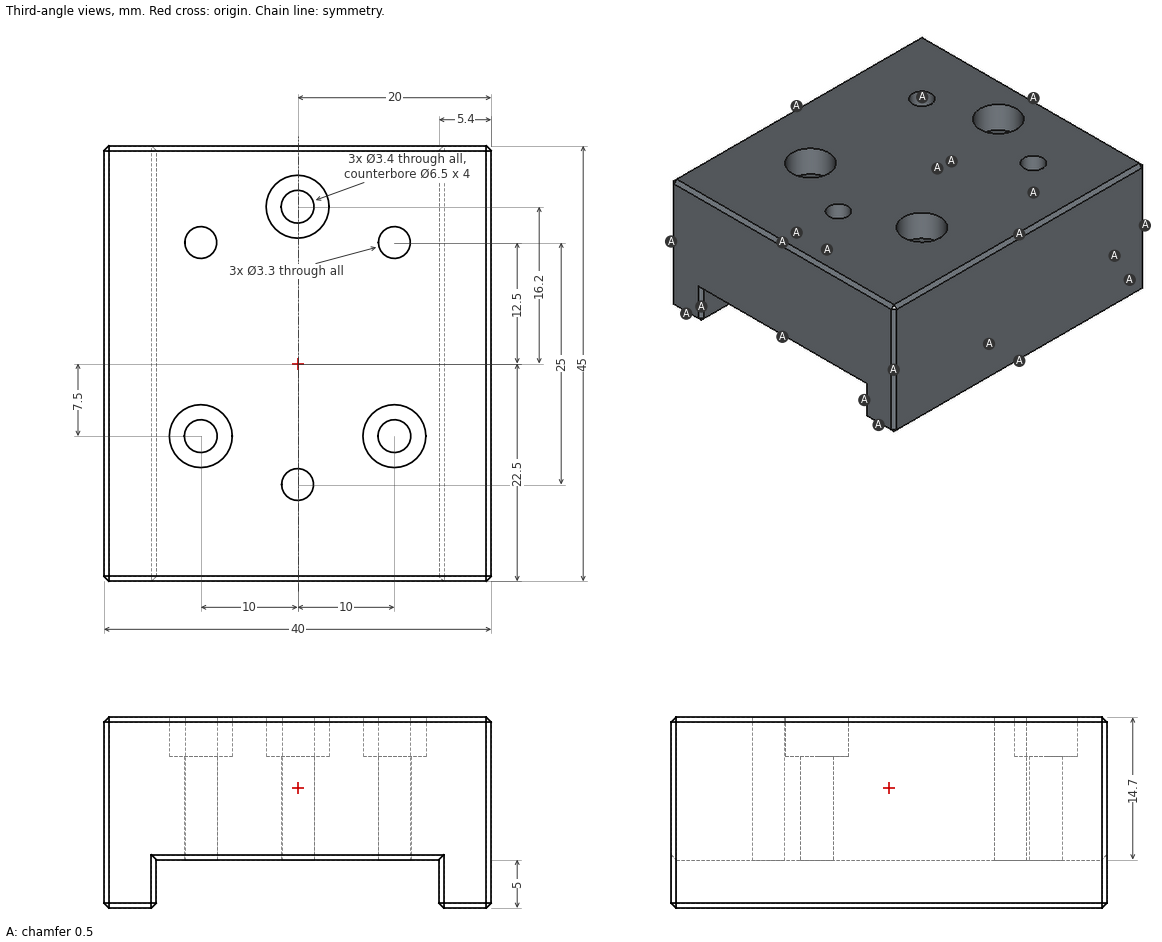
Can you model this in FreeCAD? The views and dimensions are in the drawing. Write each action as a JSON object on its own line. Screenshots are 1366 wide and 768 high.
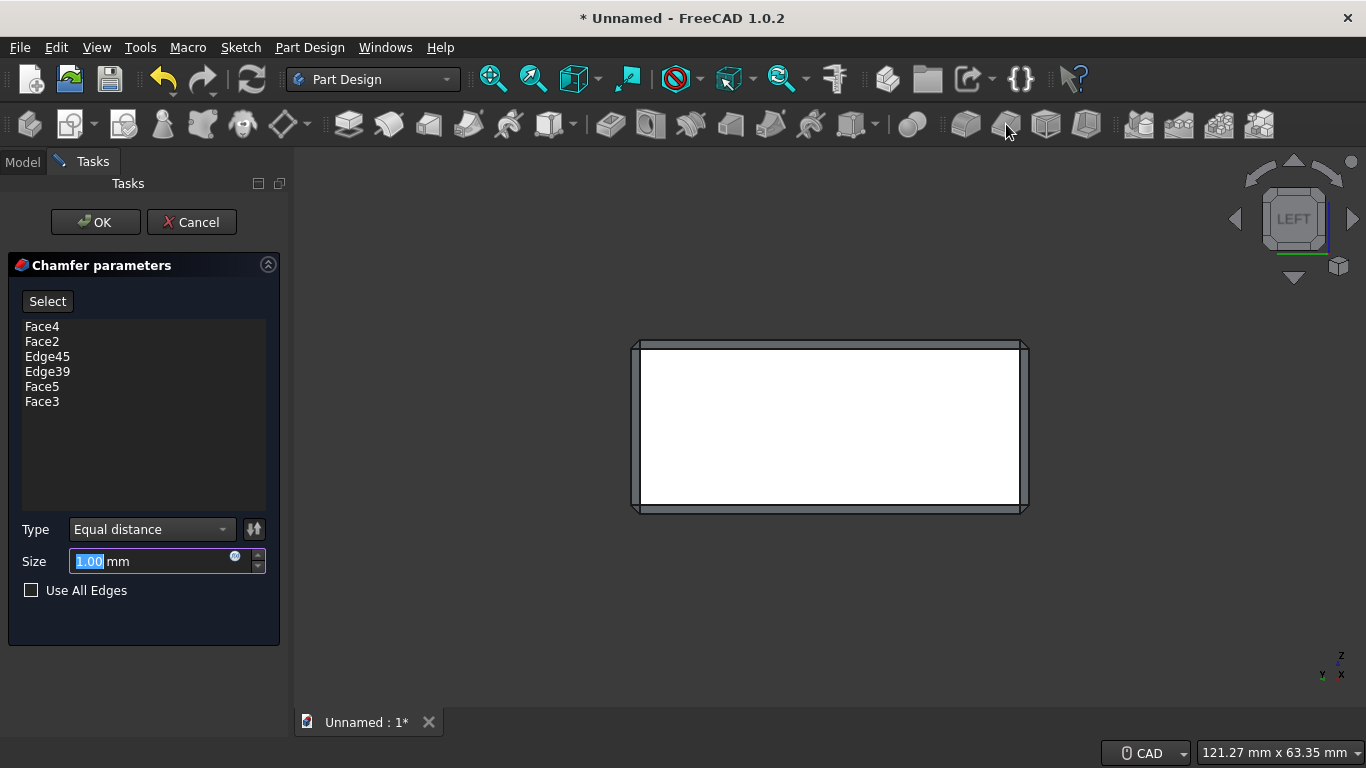
{"action": "type", "text": "0.5"}
{"action": "key", "text": "Tab"}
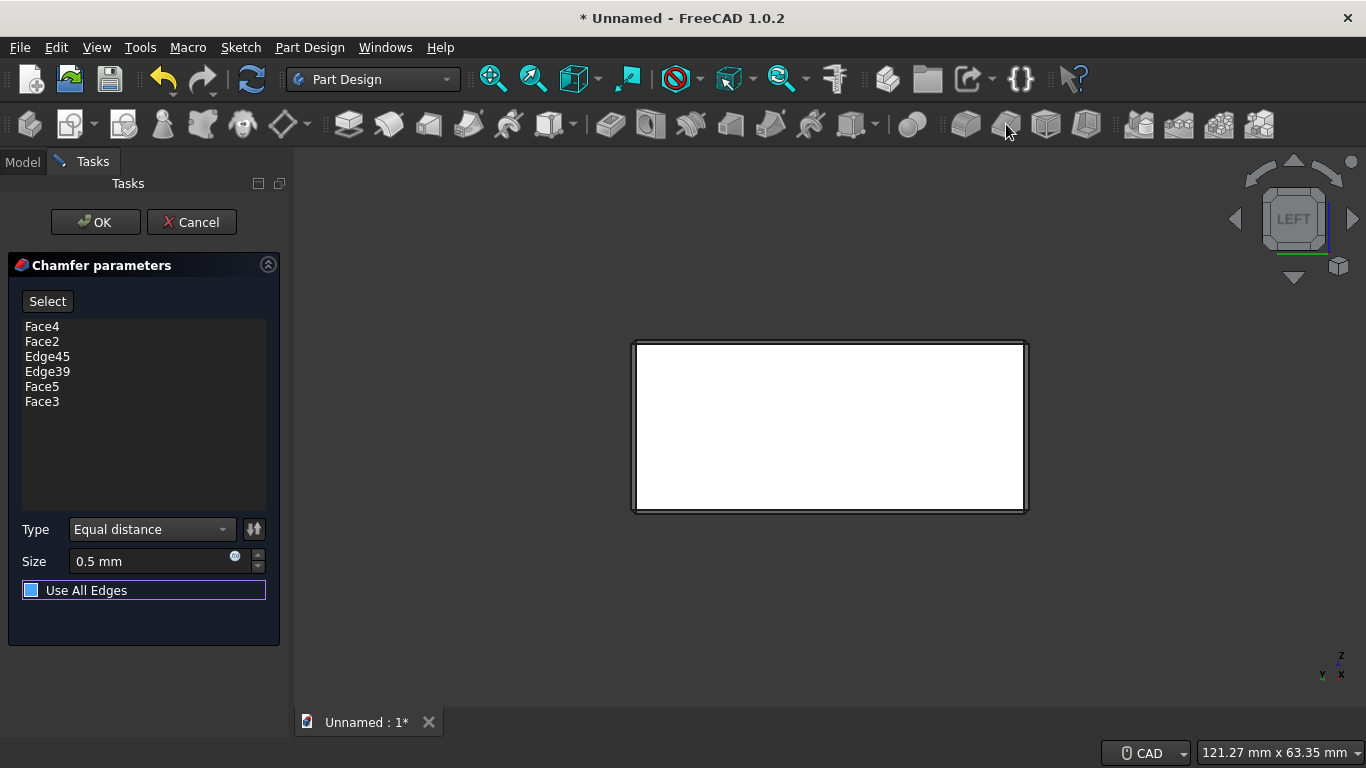
{"action": "left_click", "coordinate": [96, 222]}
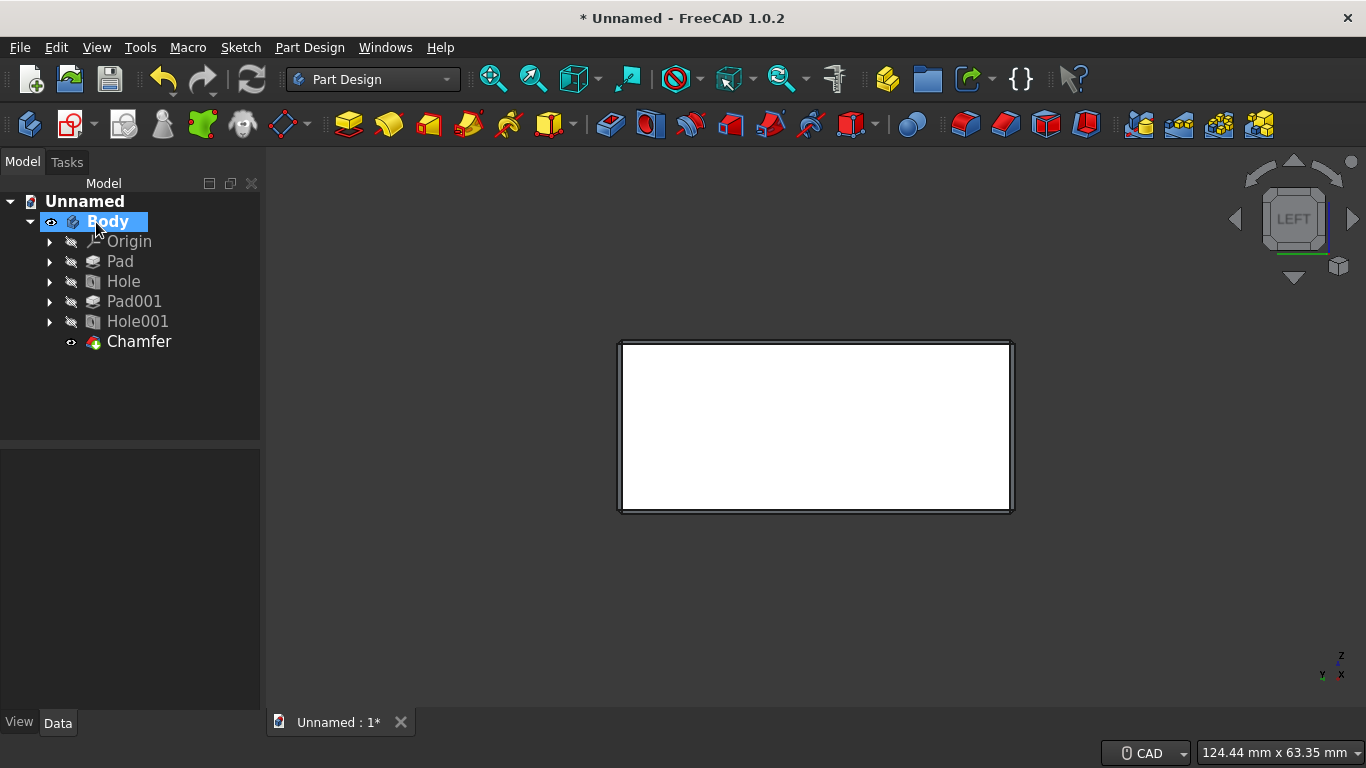
{"action": "key", "text": "0"}